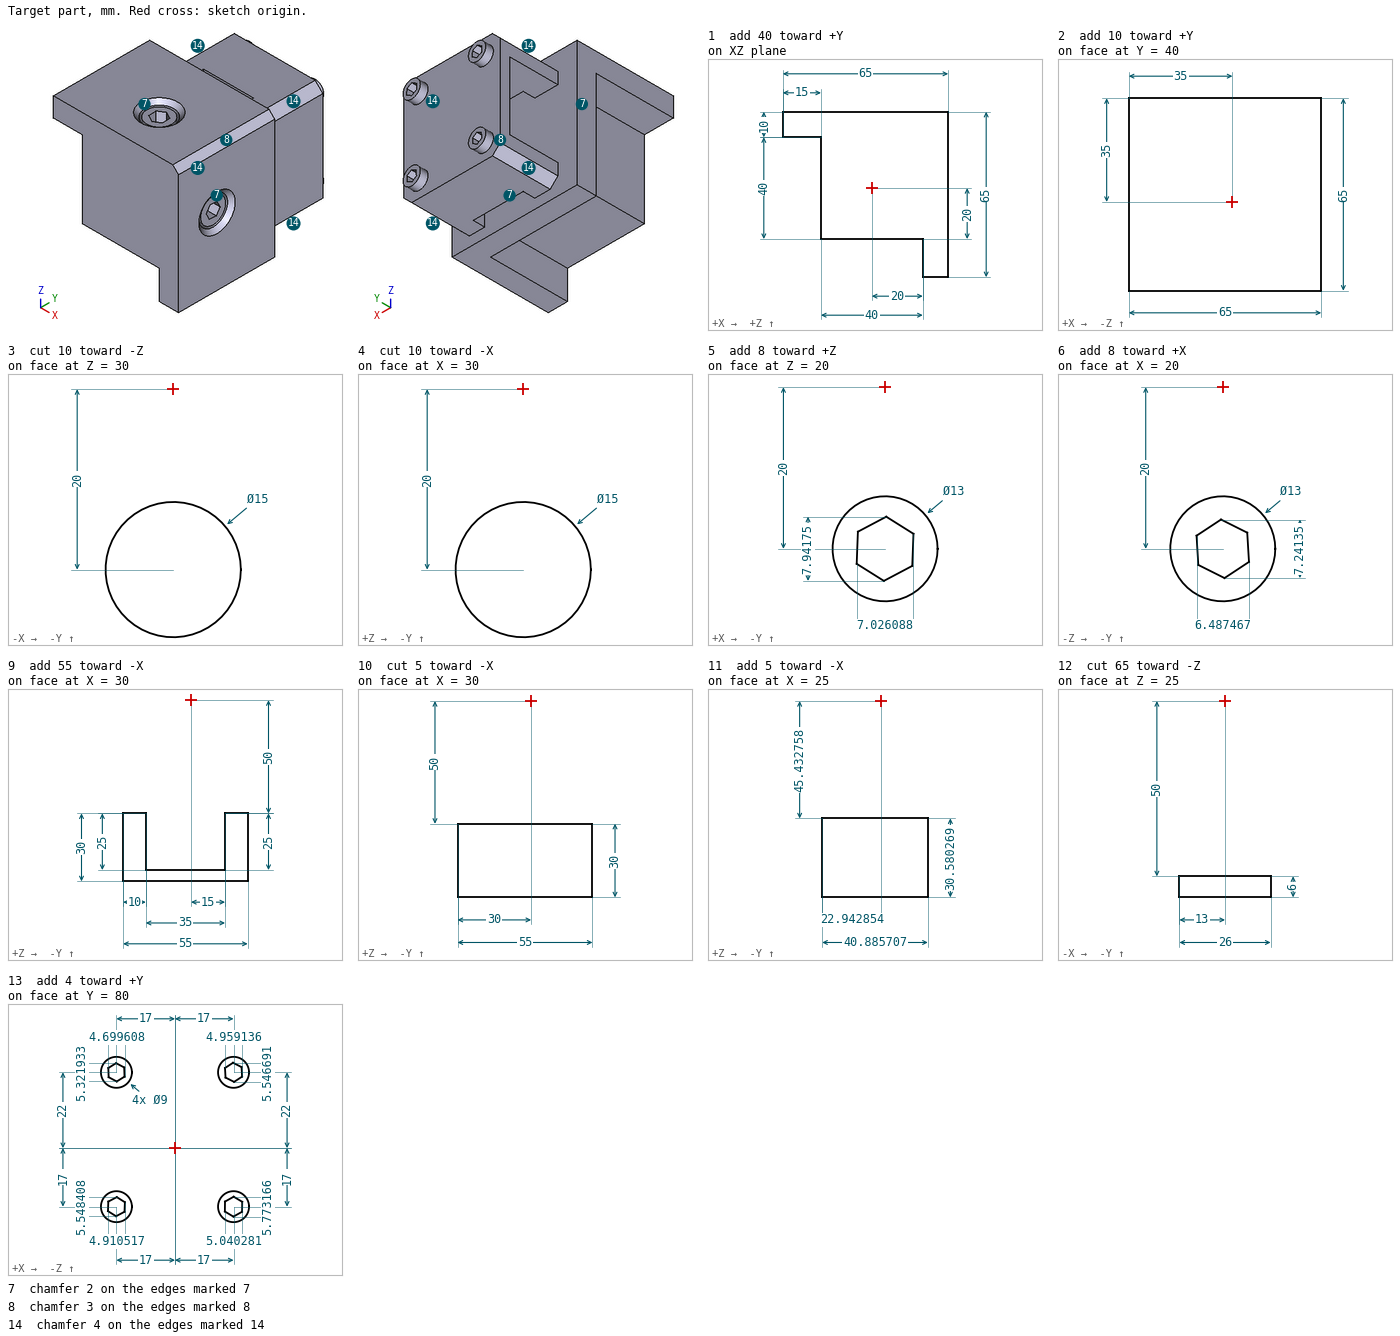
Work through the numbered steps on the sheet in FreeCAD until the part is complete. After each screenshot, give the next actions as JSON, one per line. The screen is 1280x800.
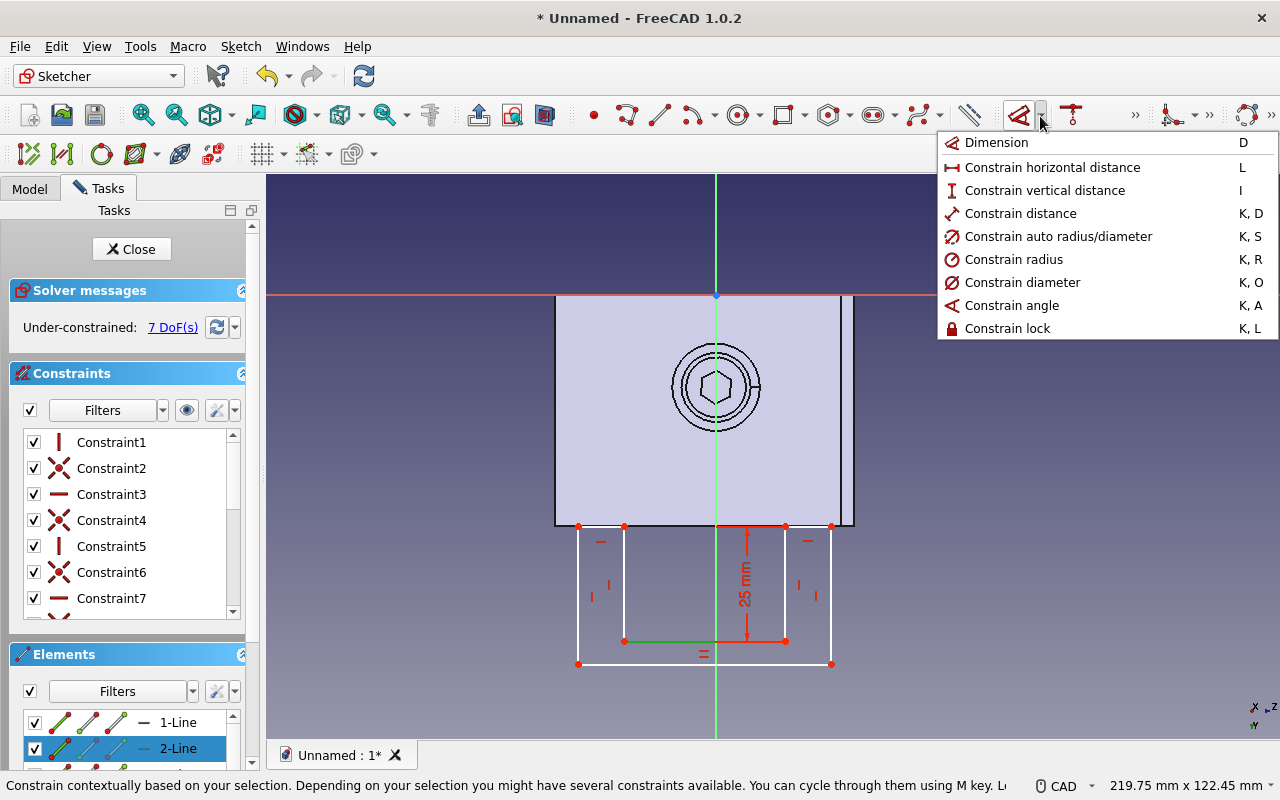
{"action": "left_click", "coordinate": [1108, 168]}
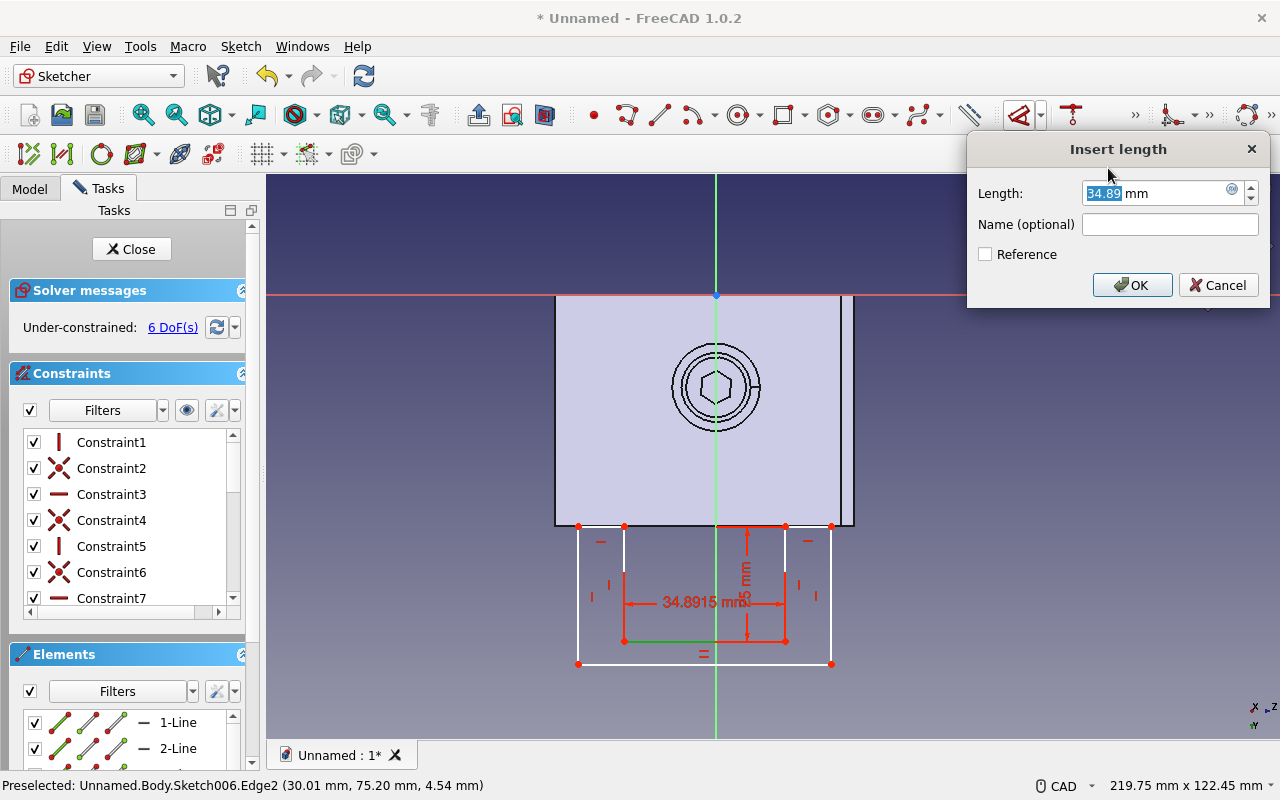
{"action": "type", "text": "35"}
{"action": "key", "text": "Return"}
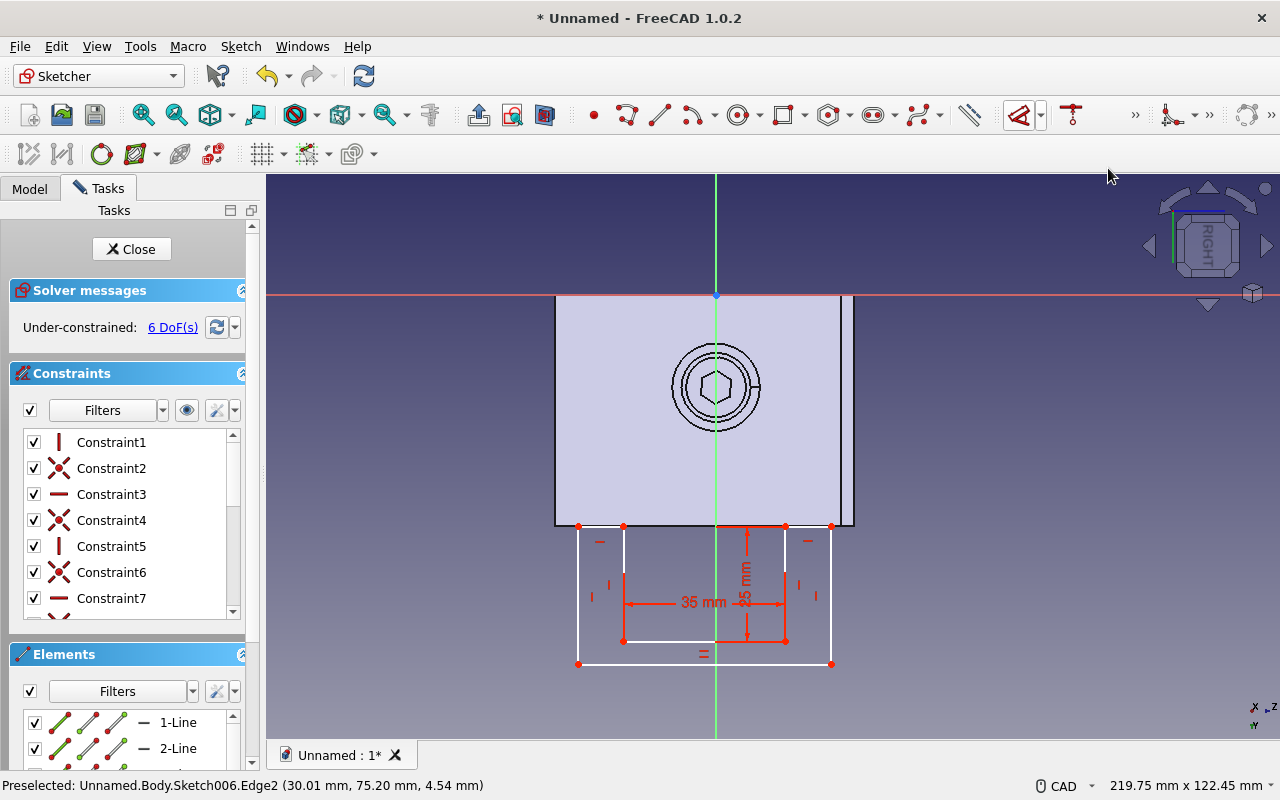
{"action": "left_click", "coordinate": [624, 608]}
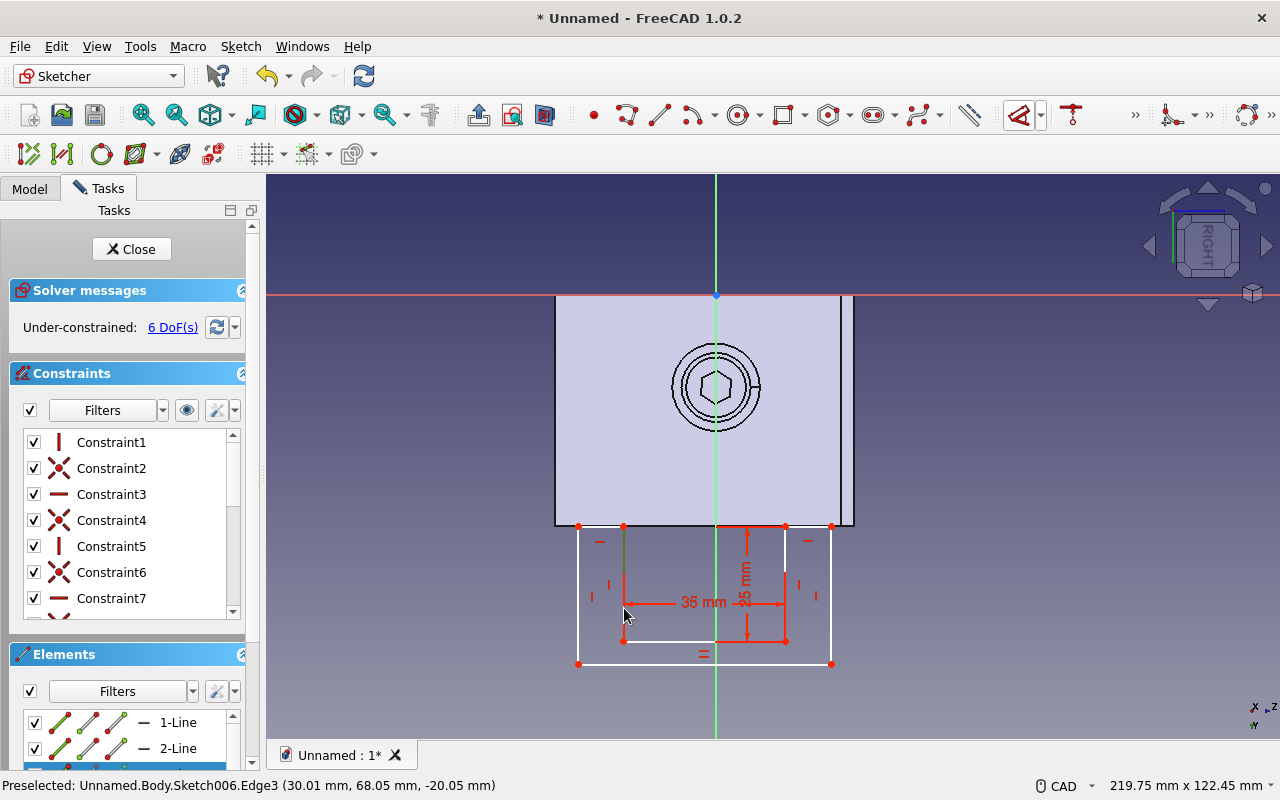
{"action": "left_click", "coordinate": [1040, 116]}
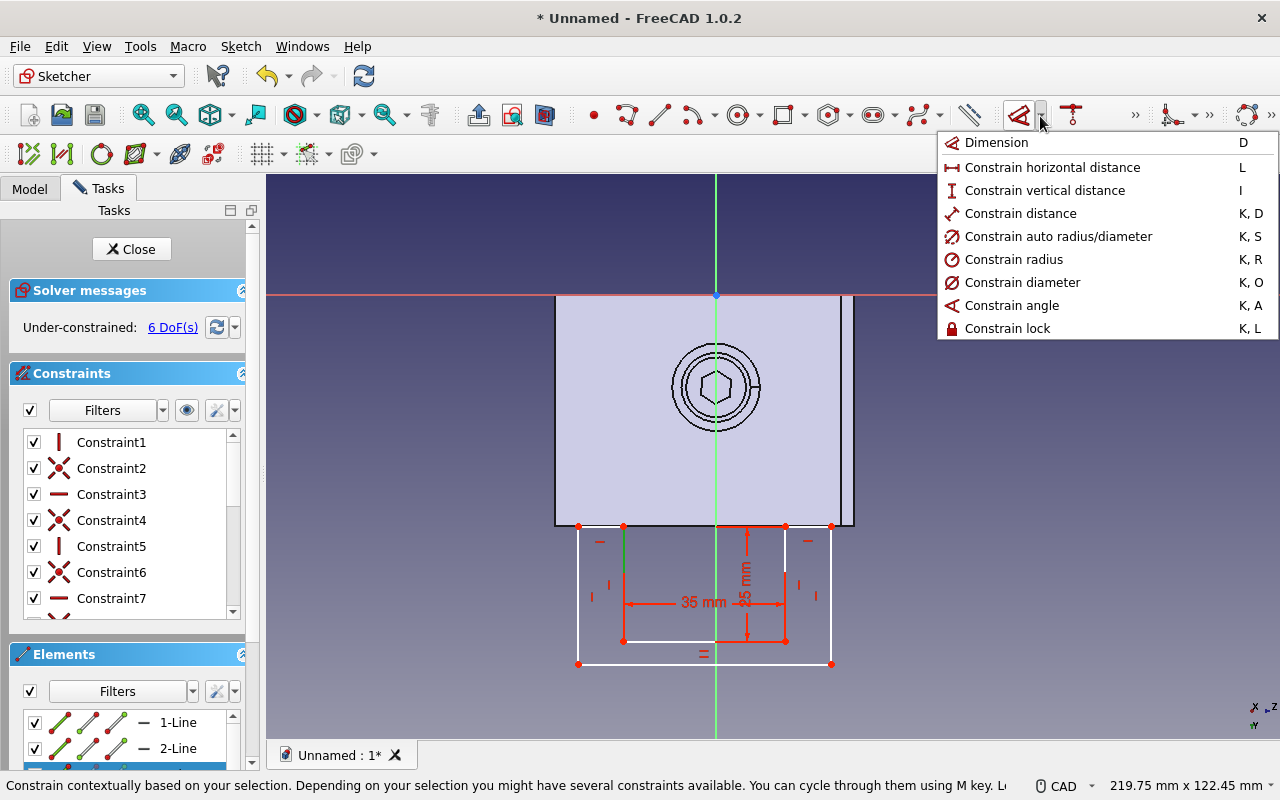
{"action": "left_click", "coordinate": [1108, 190]}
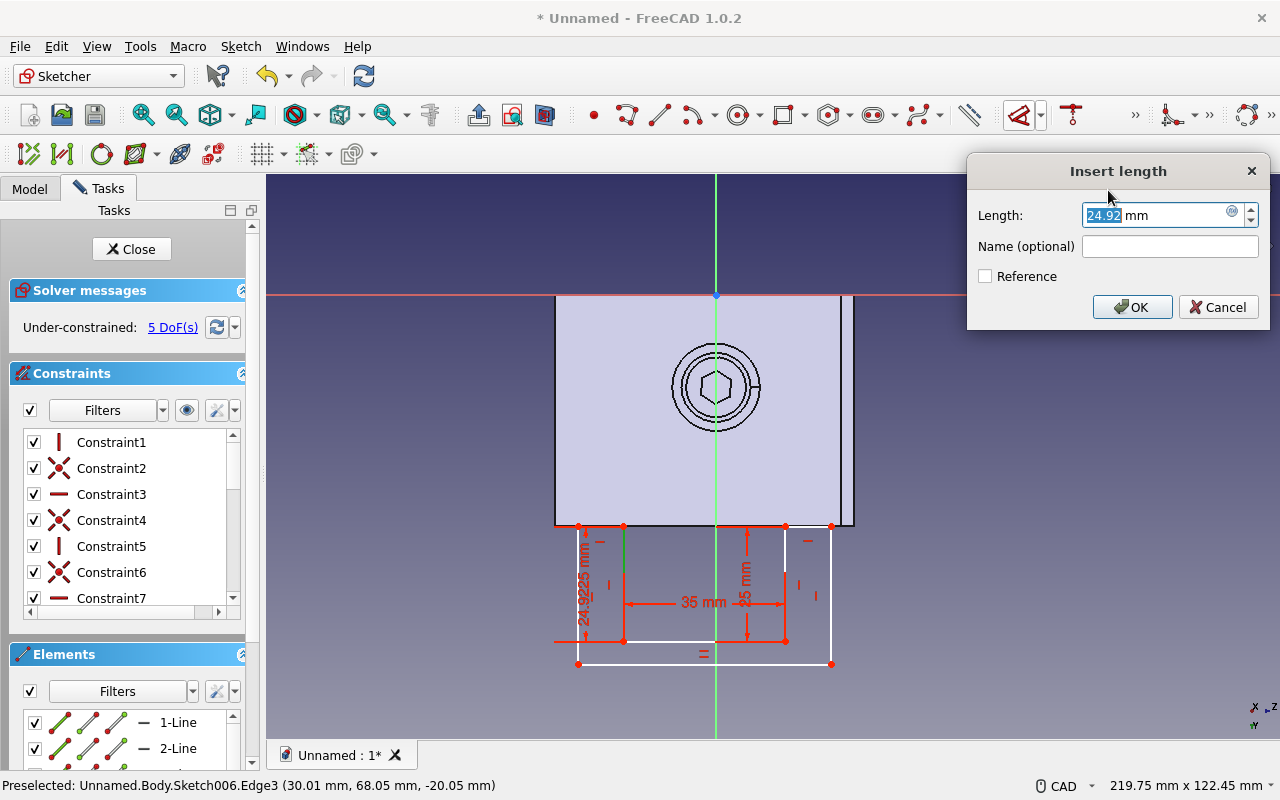
{"action": "type", "text": "25"}
{"action": "key", "text": "Return"}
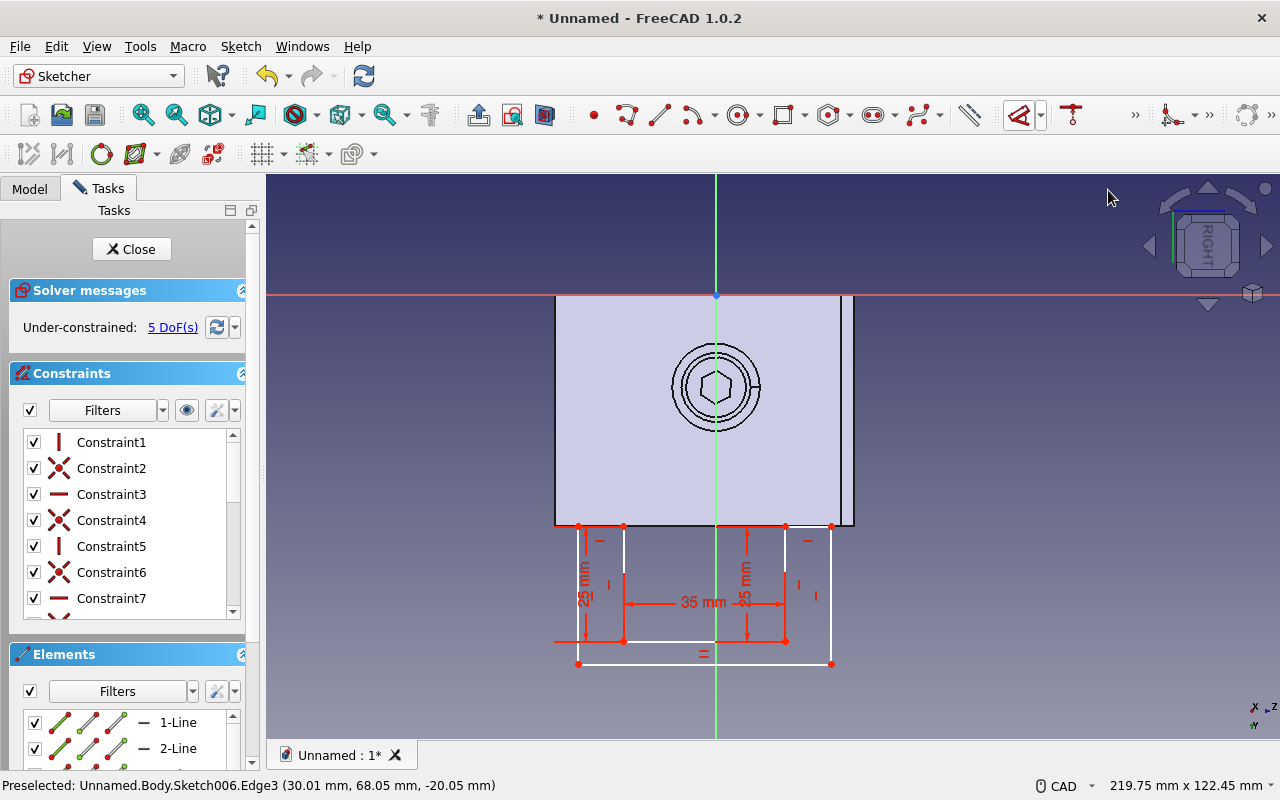
{"action": "left_click", "coordinate": [610, 527]}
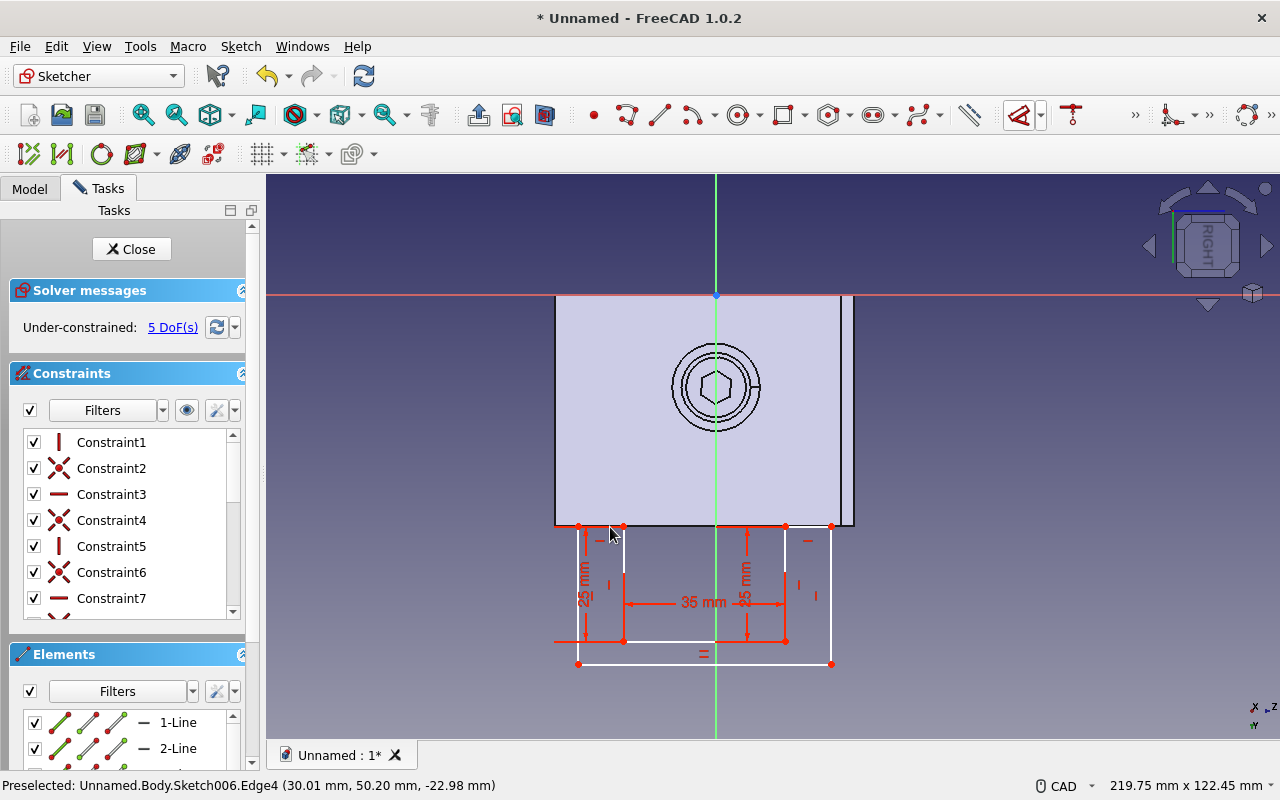
{"action": "left_click", "coordinate": [1040, 116]}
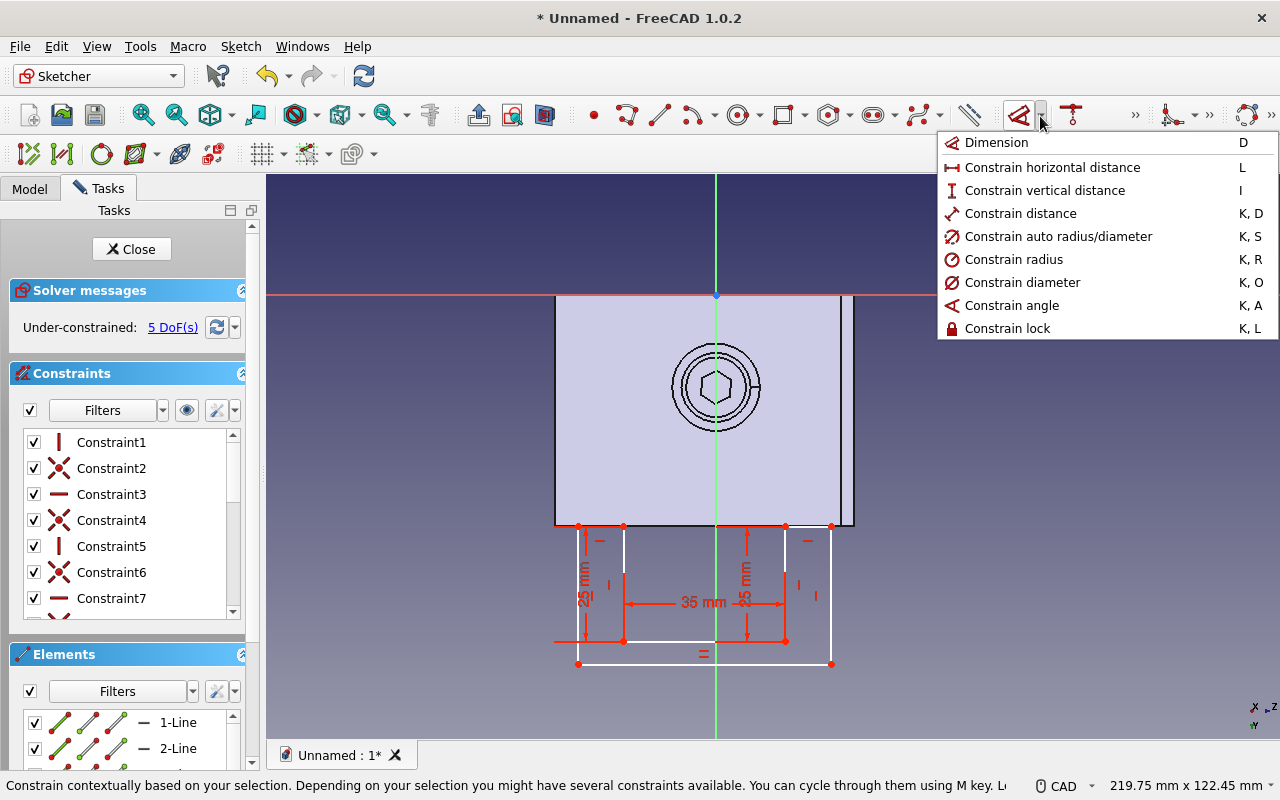
{"action": "left_click", "coordinate": [1108, 168]}